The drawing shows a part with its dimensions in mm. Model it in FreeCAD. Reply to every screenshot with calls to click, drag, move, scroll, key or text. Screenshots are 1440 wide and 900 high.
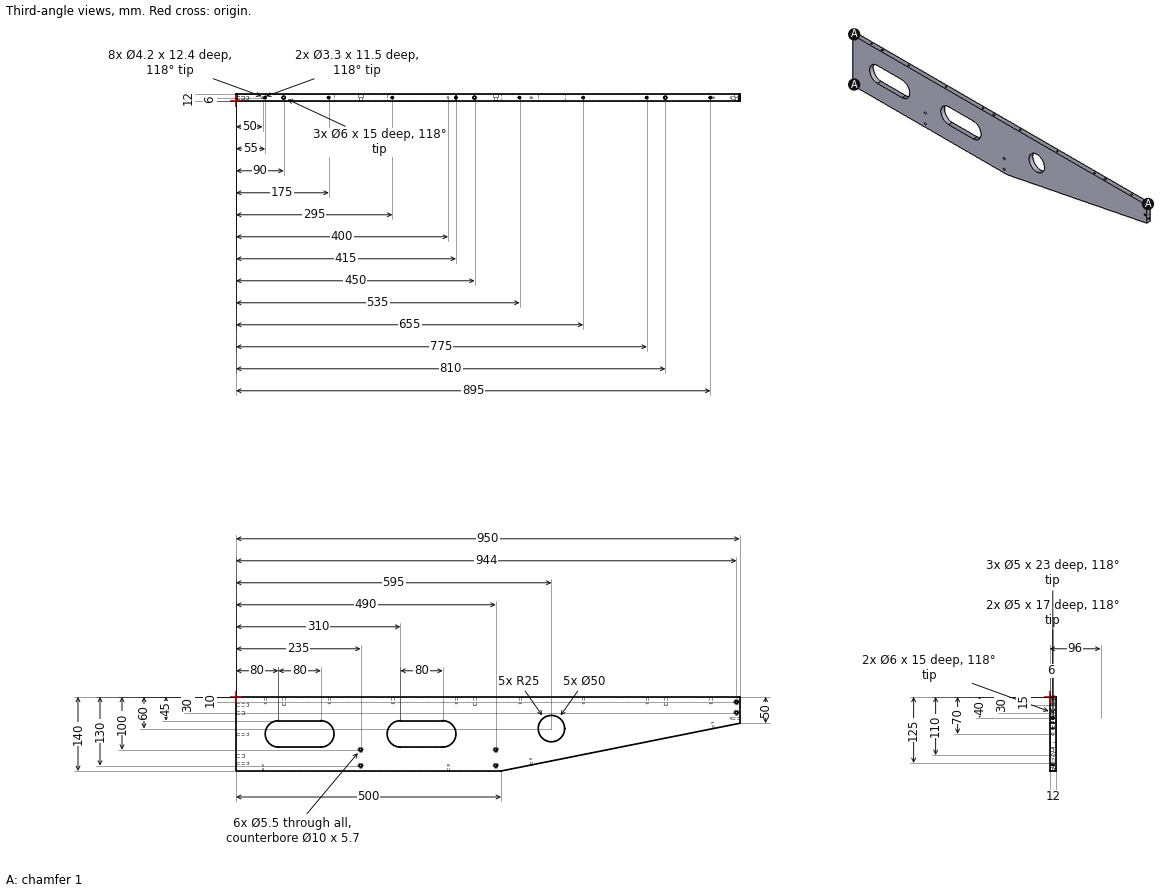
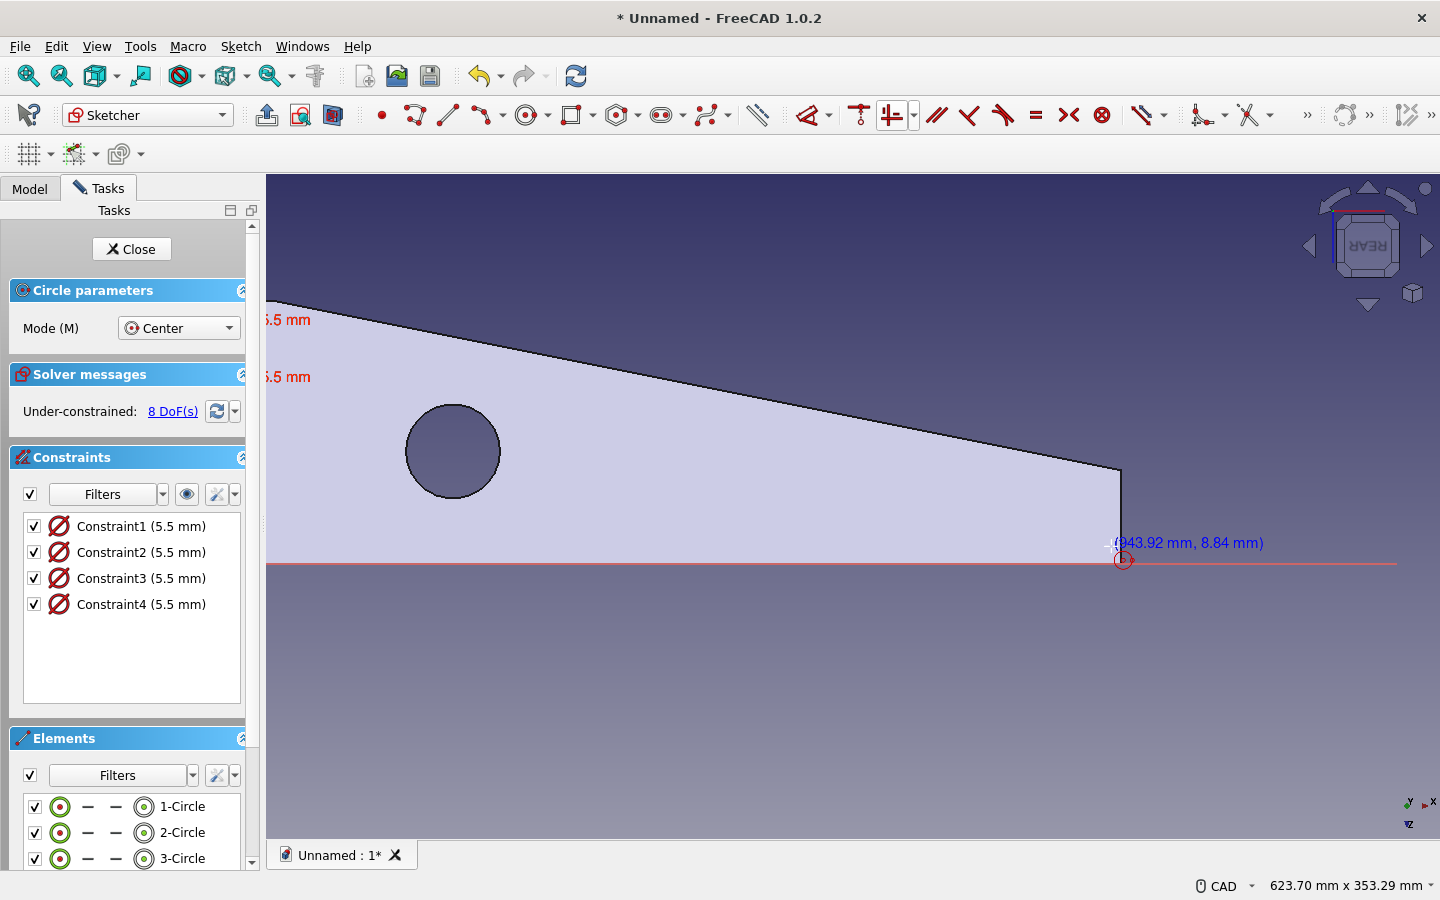
click(1110, 546)
move(1114, 542)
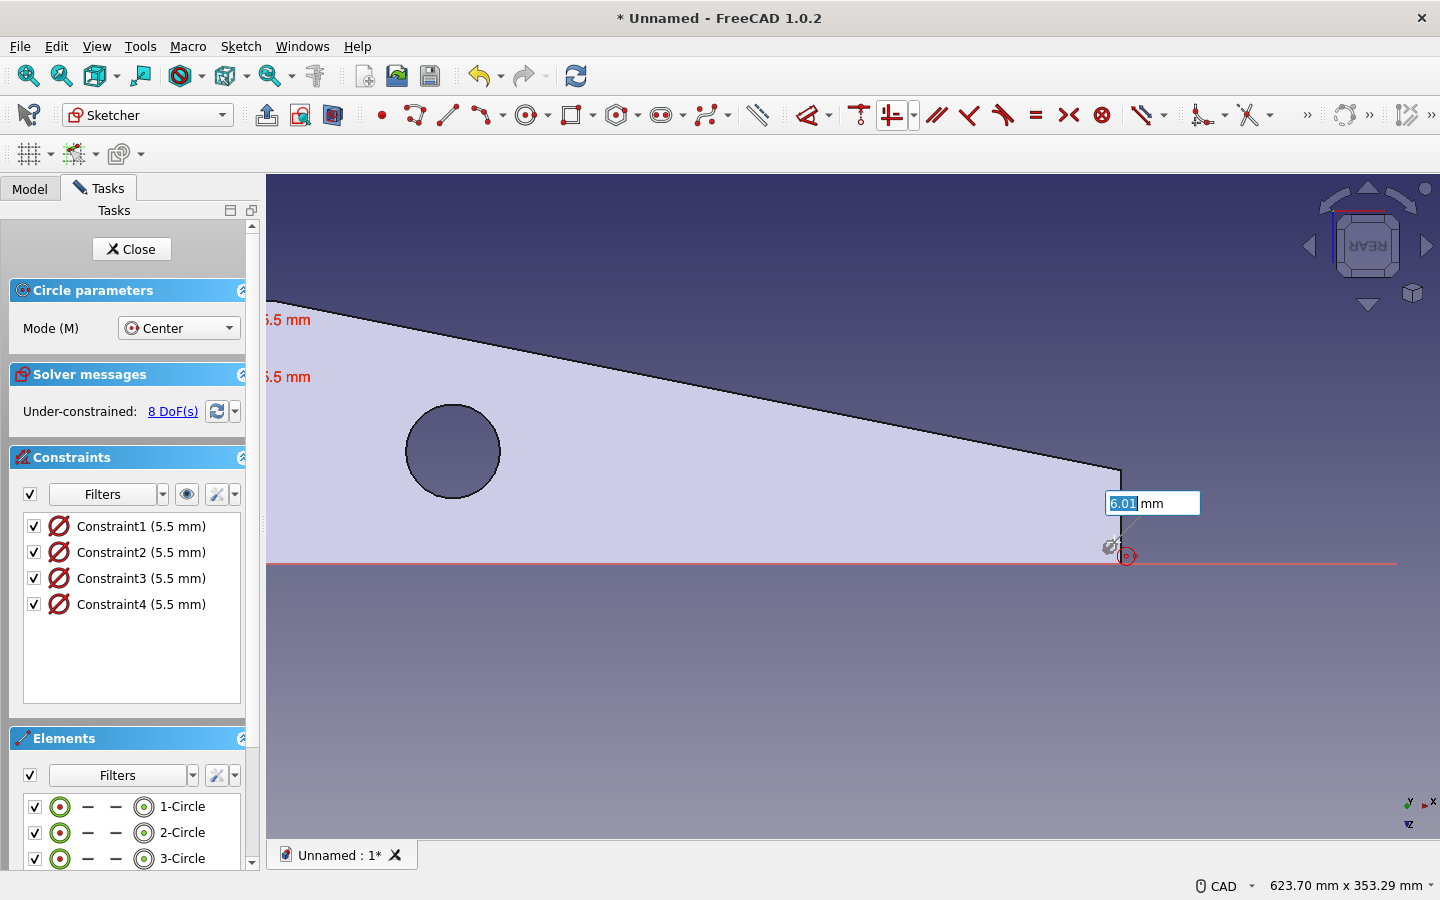
text(5.5)
key(Return)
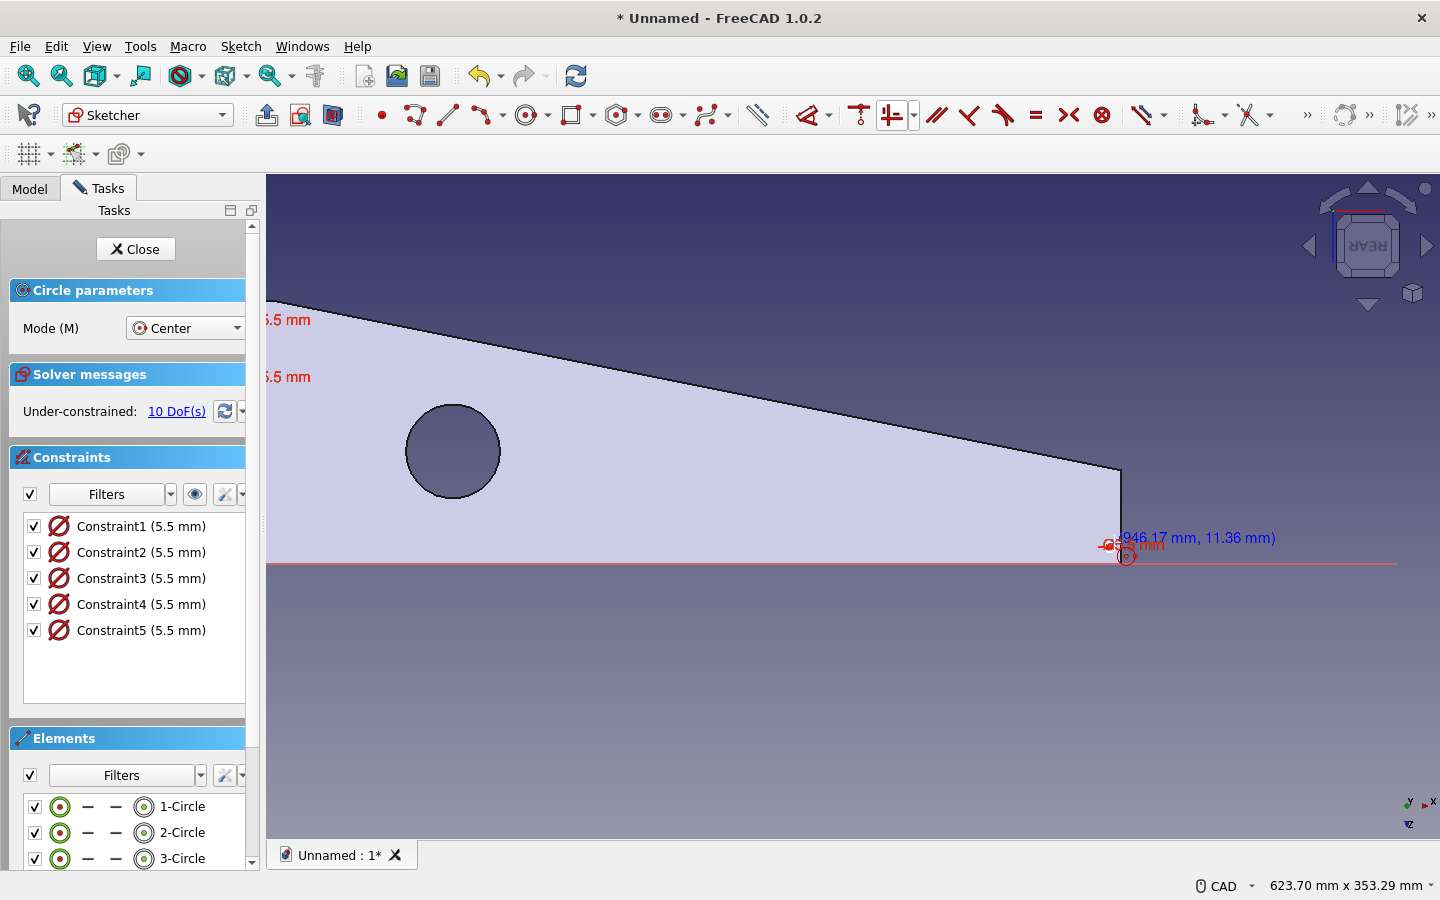
scroll(1110, 508, up, 8)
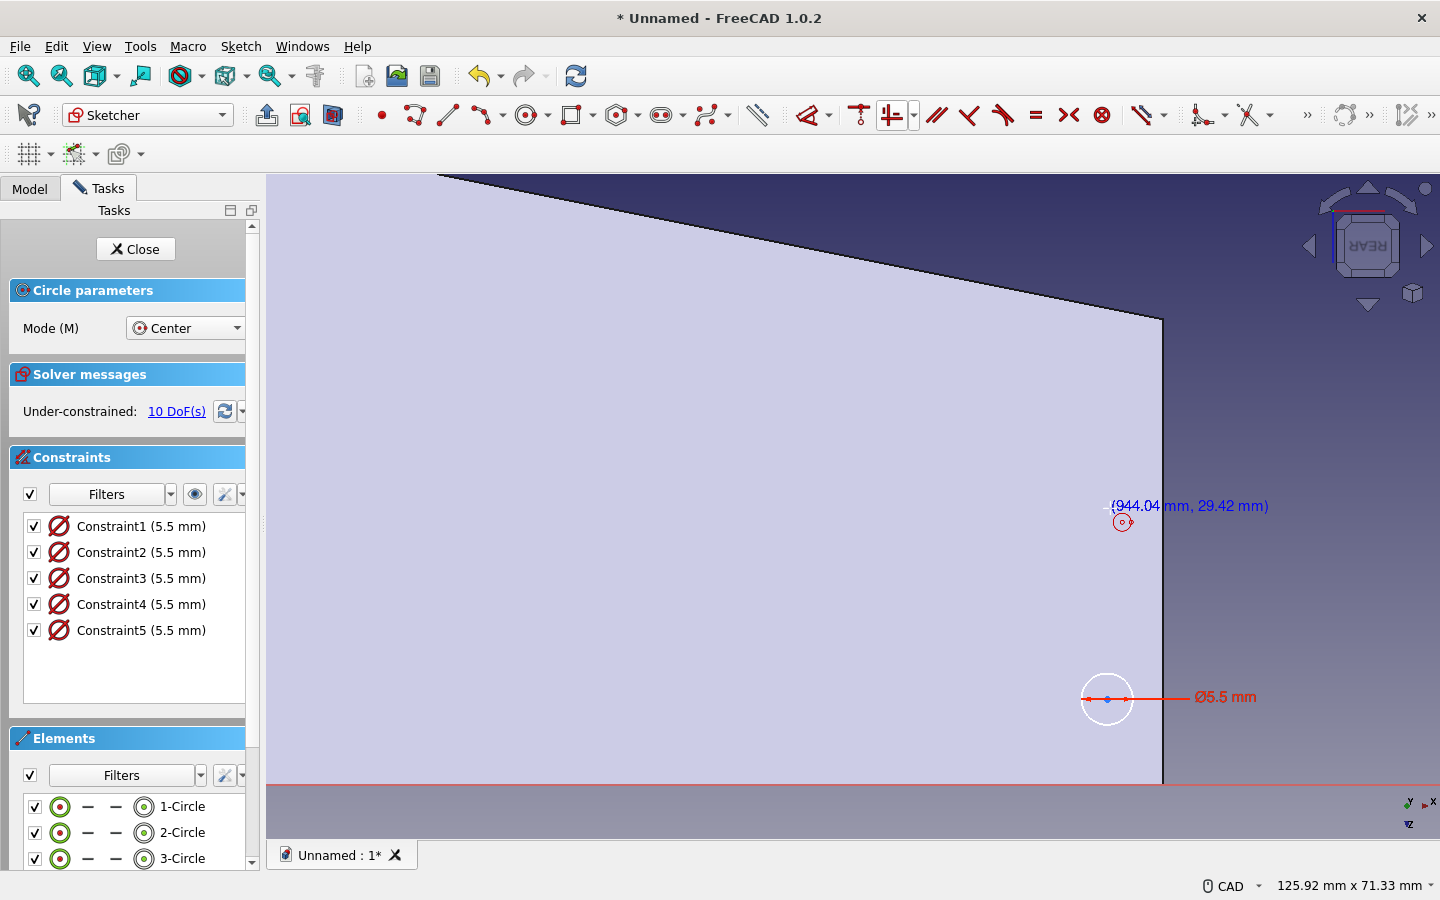
scroll(1111, 534, down, 13)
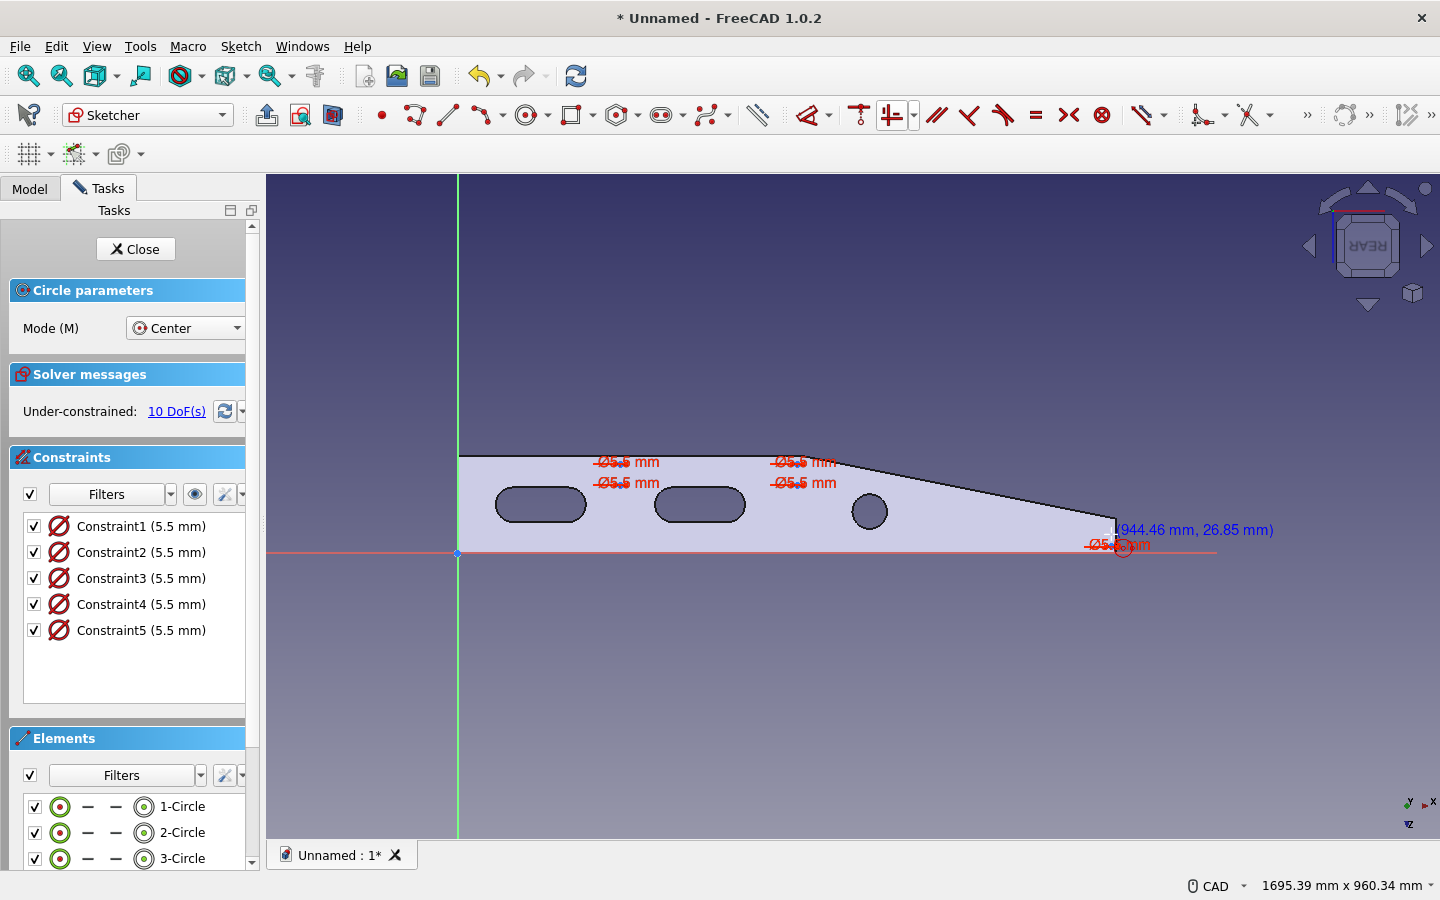
scroll(1111, 532, up, 2)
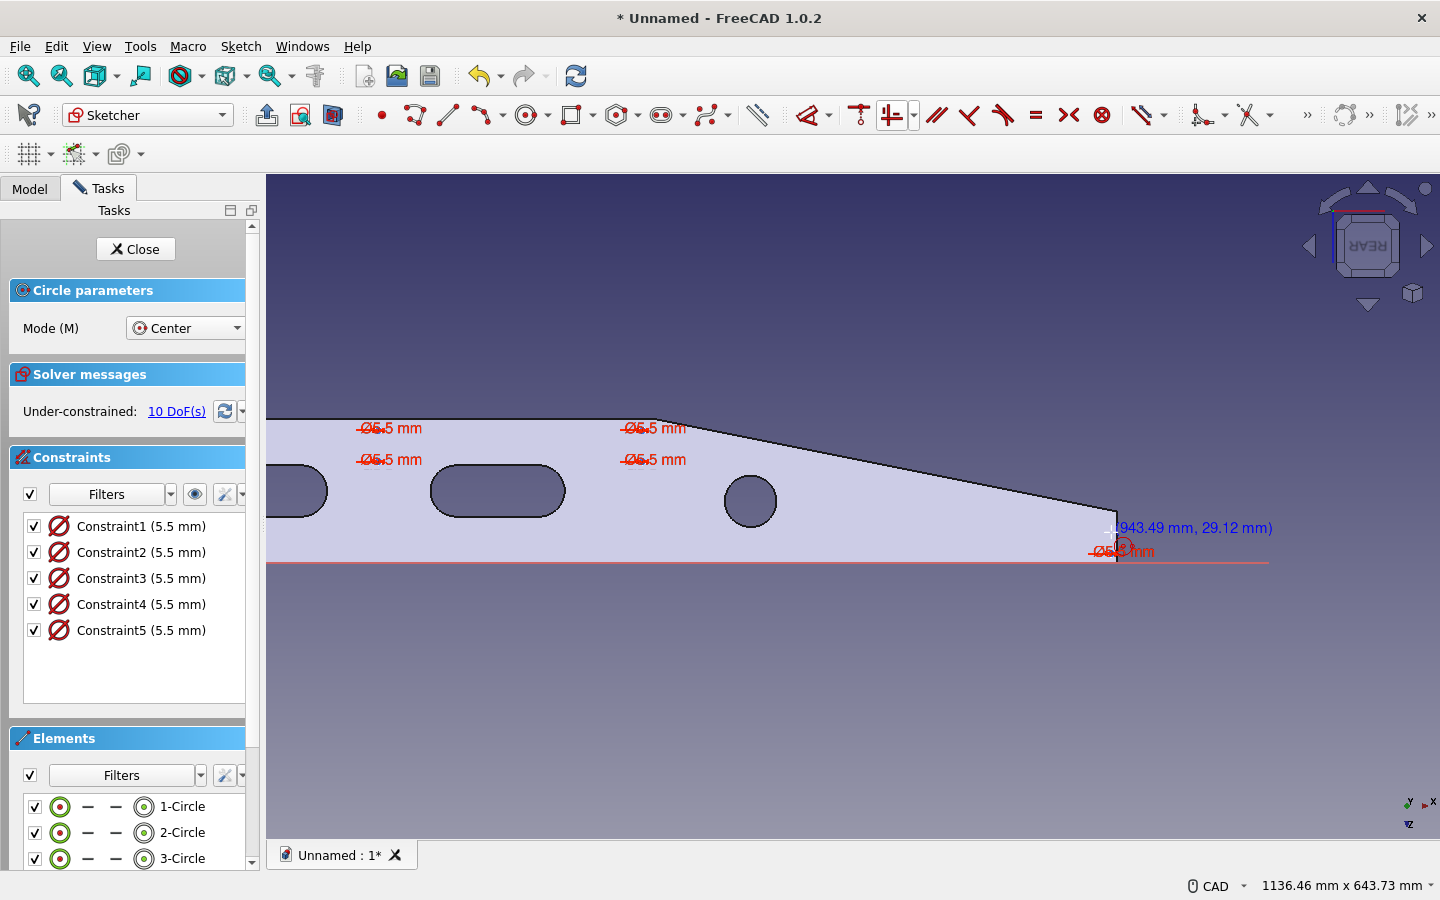
click(1111, 532)
move(1113, 530)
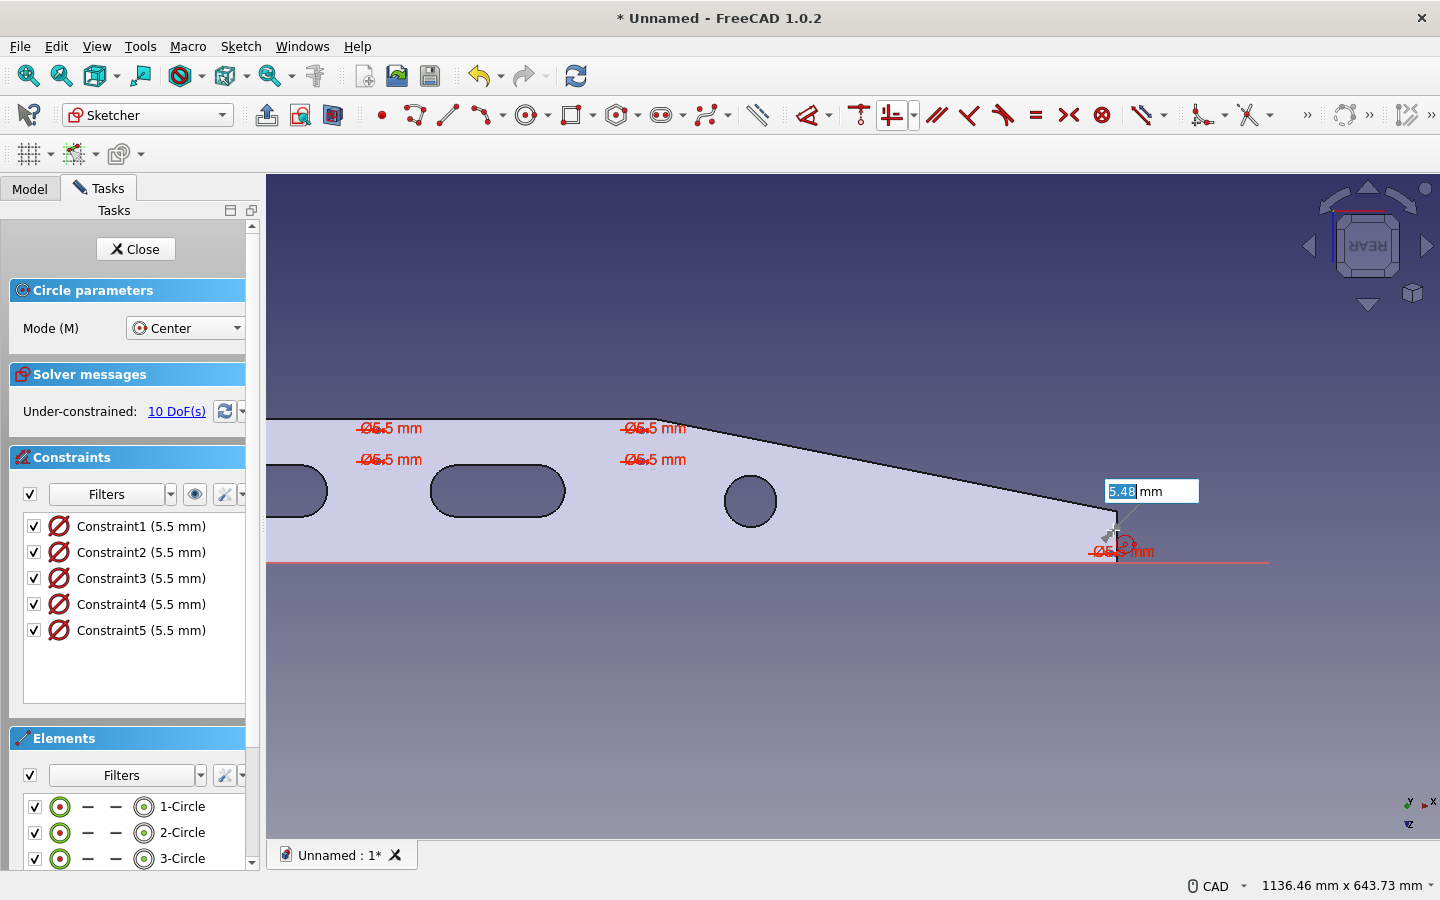
text(5.5)
key(Return)
key(Escape)